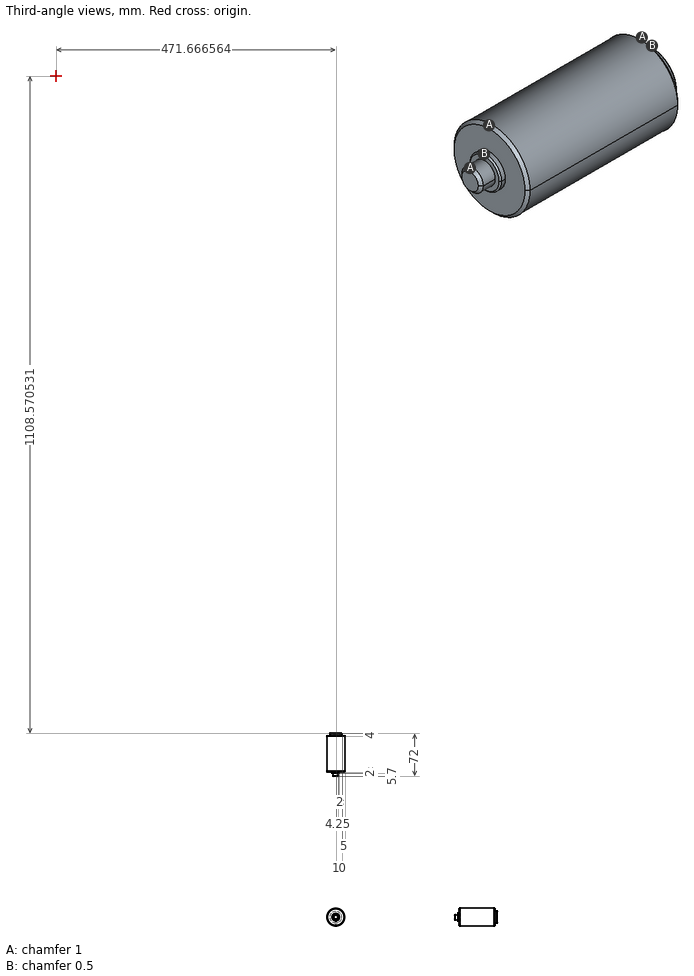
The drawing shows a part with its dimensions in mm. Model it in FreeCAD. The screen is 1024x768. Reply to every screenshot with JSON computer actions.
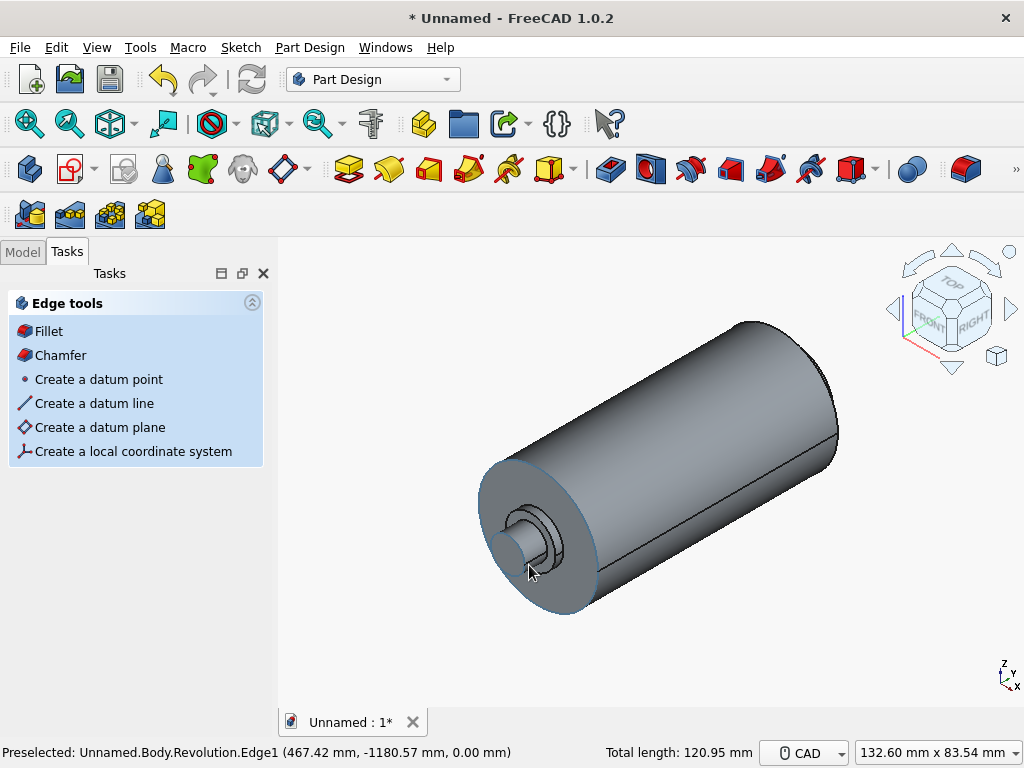
{"action": "left_click", "coordinate": [797, 343], "text": "ctrl"}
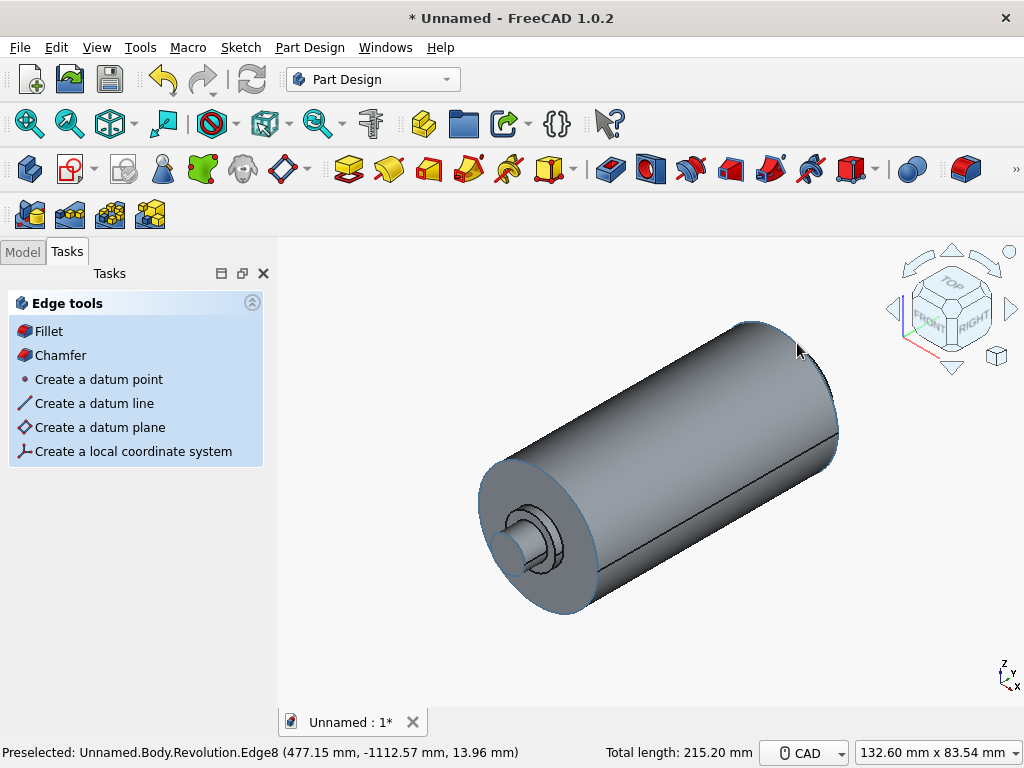
{"action": "left_click", "coordinate": [136, 355]}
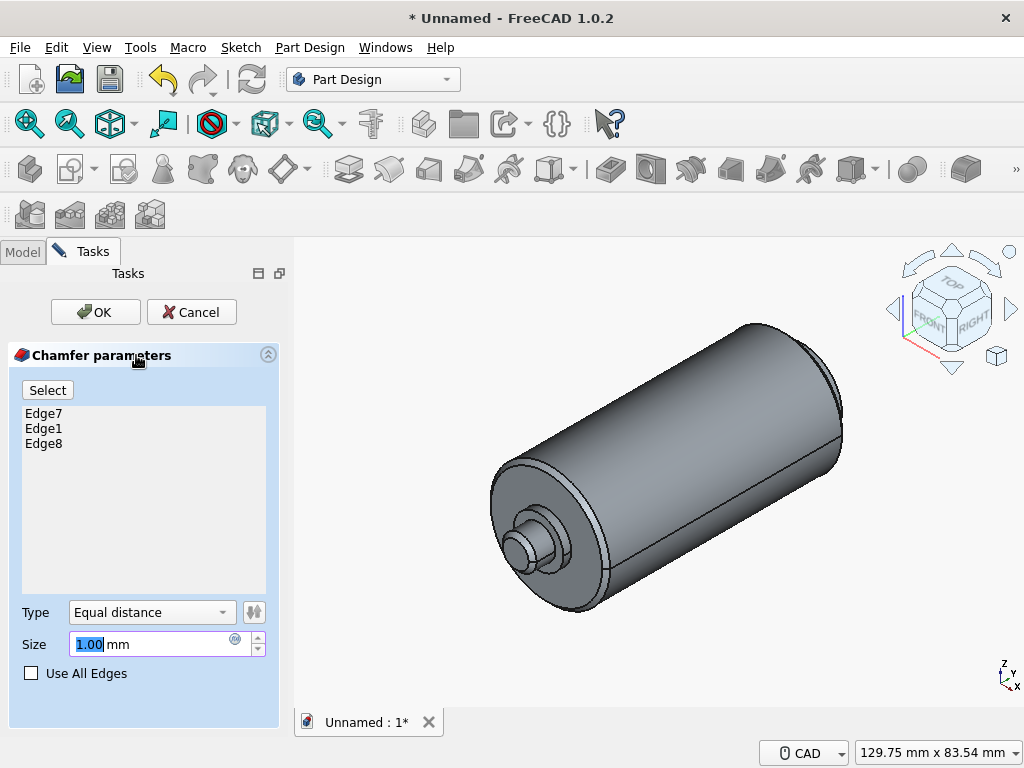
{"action": "type", "text": "1"}
{"action": "key", "text": "Tab"}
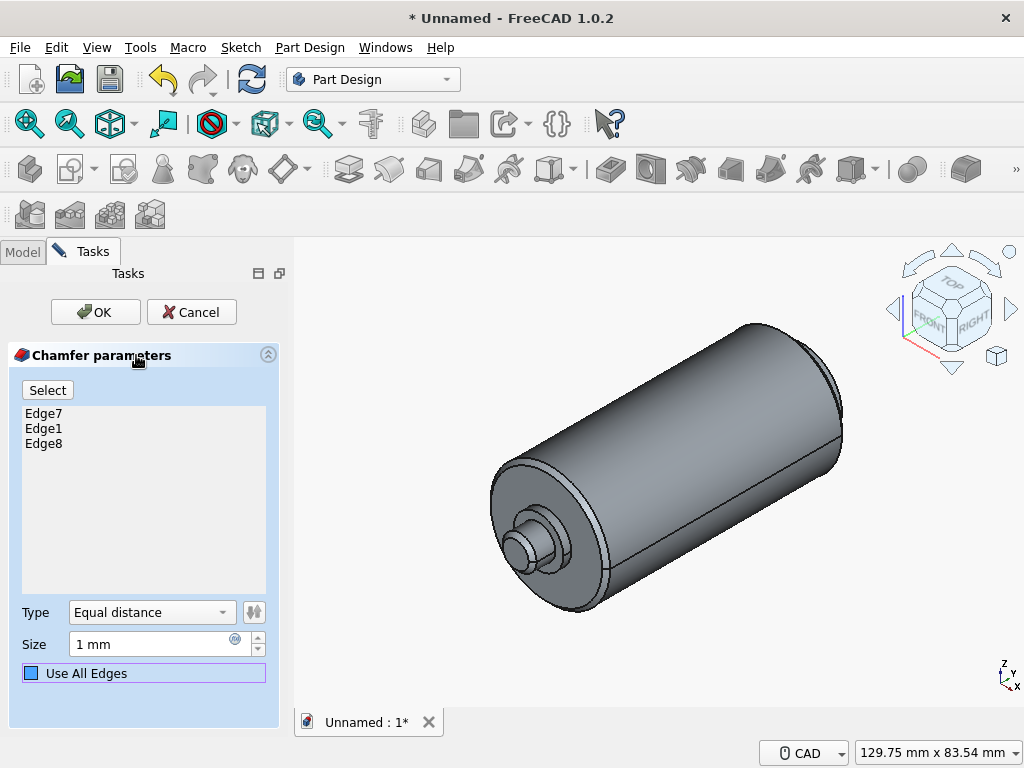
{"action": "left_click", "coordinate": [96, 312]}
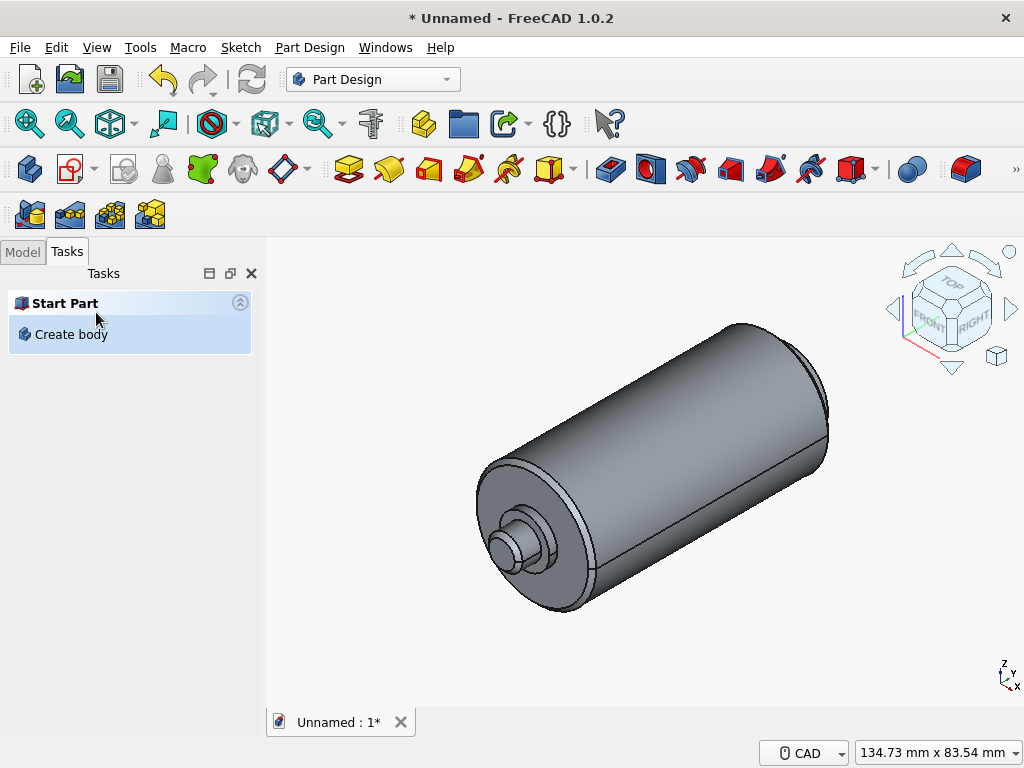
{"action": "left_click", "coordinate": [517, 509]}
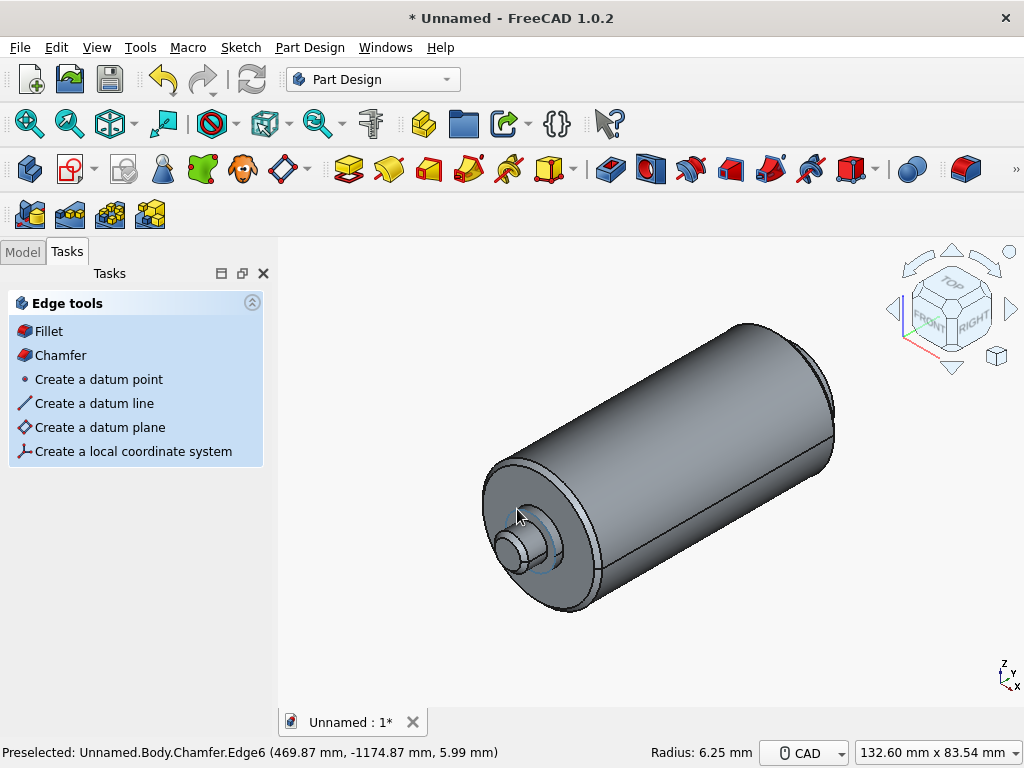
{"action": "key", "text": "2"}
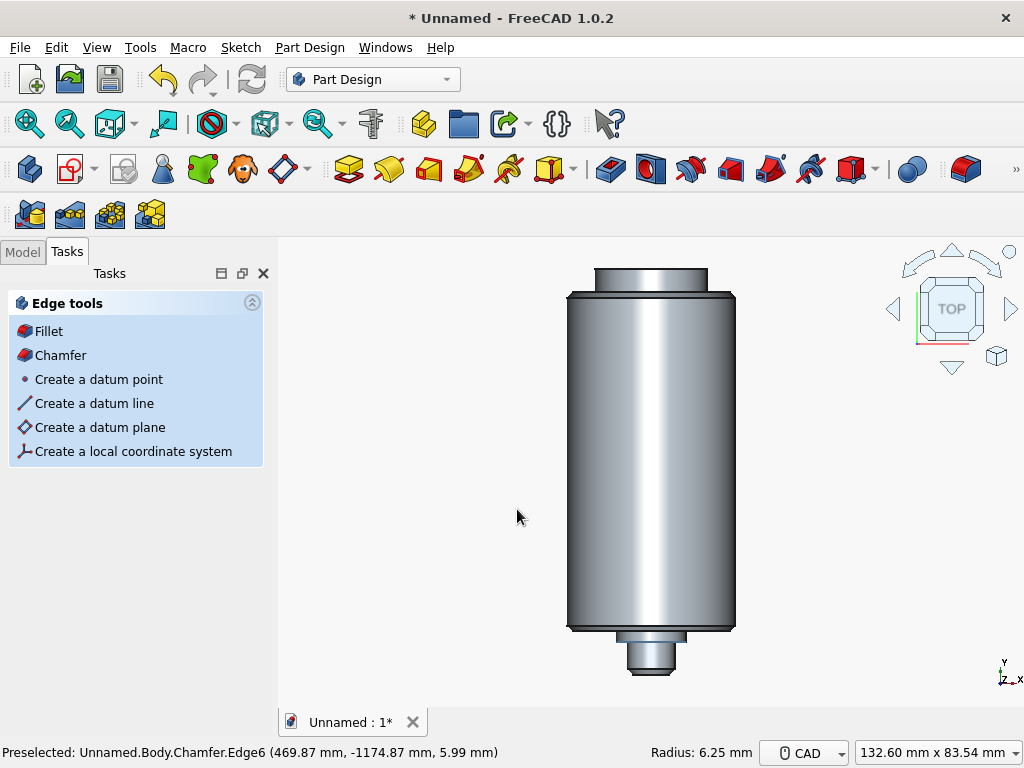
{"action": "left_click", "coordinate": [605, 268], "text": "ctrl"}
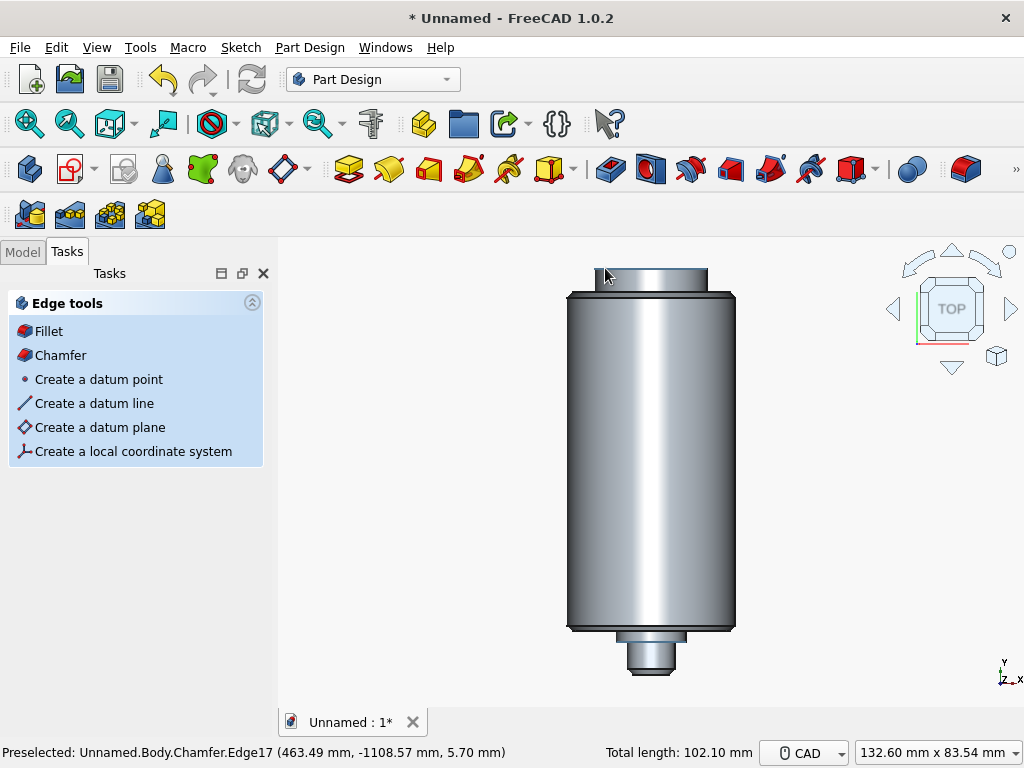
{"action": "left_click", "coordinate": [136, 355]}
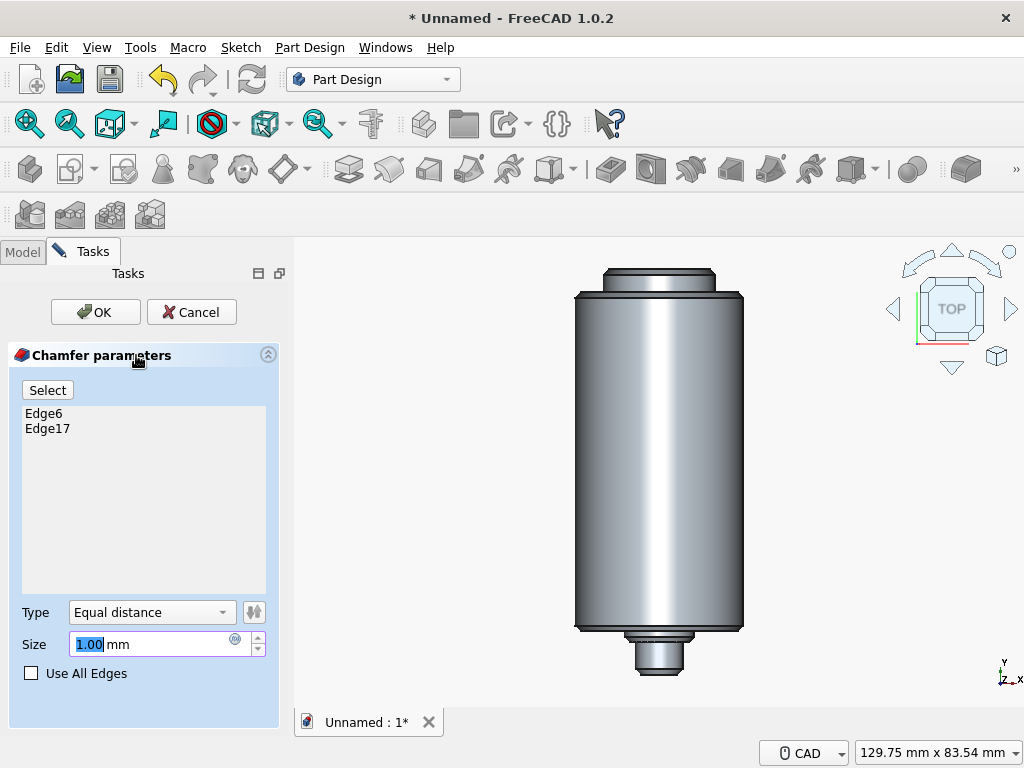
{"action": "type", "text": "0.5"}
{"action": "key", "text": "Tab"}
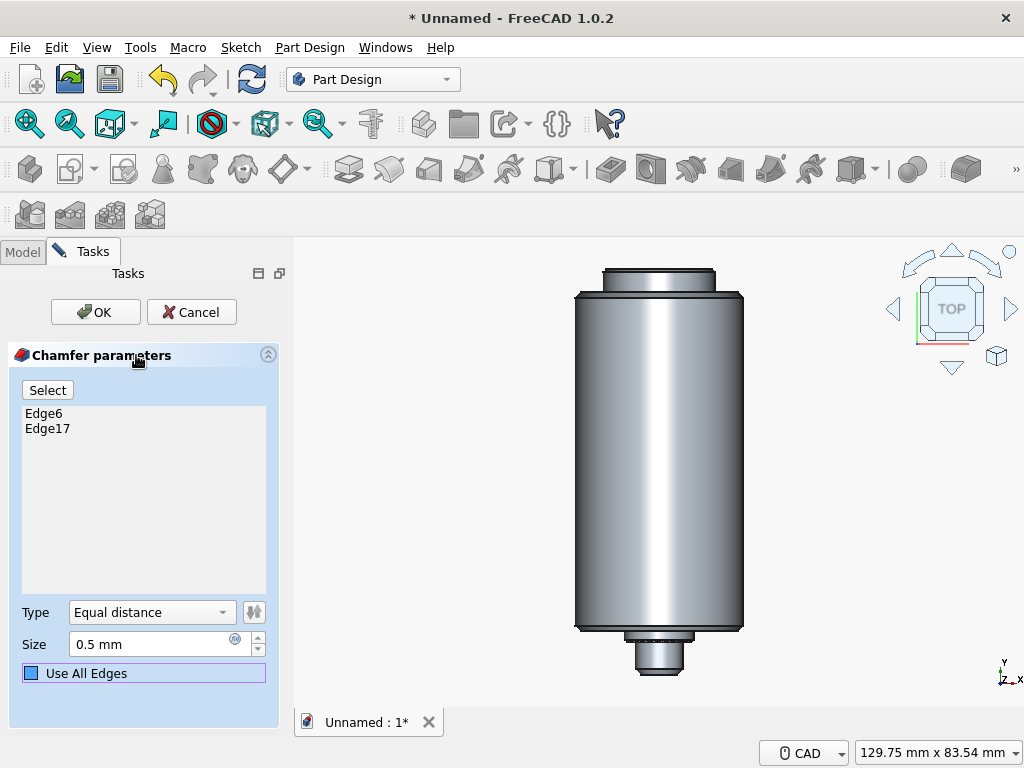
{"action": "left_click", "coordinate": [96, 312]}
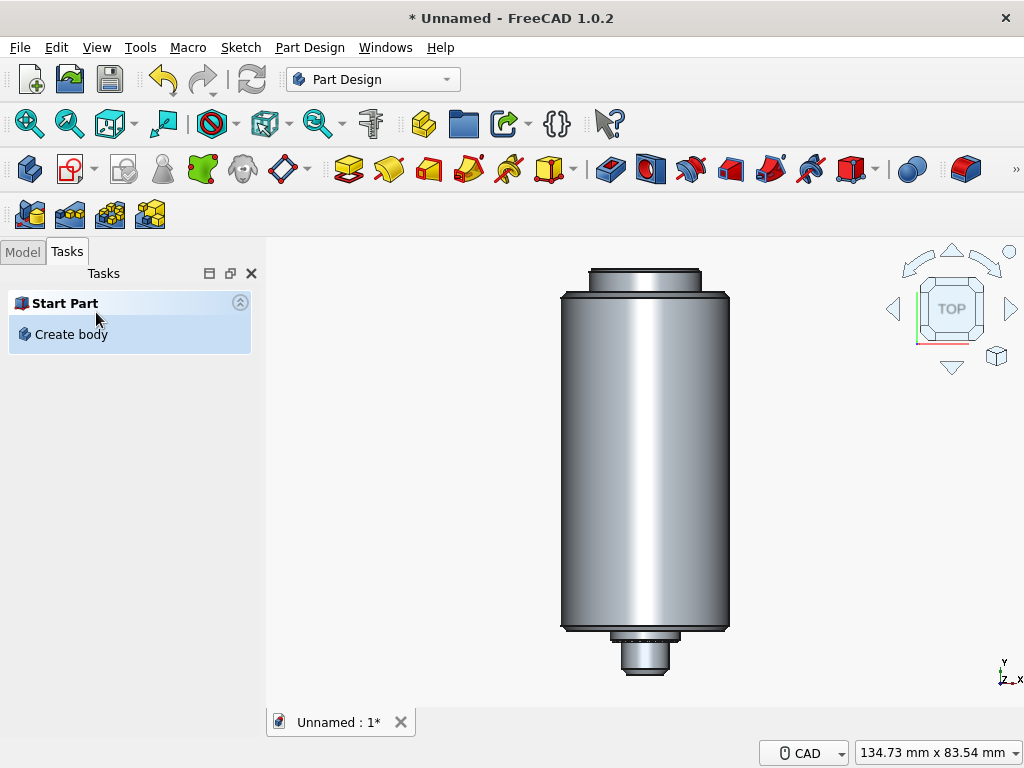
{"action": "key", "text": "0"}